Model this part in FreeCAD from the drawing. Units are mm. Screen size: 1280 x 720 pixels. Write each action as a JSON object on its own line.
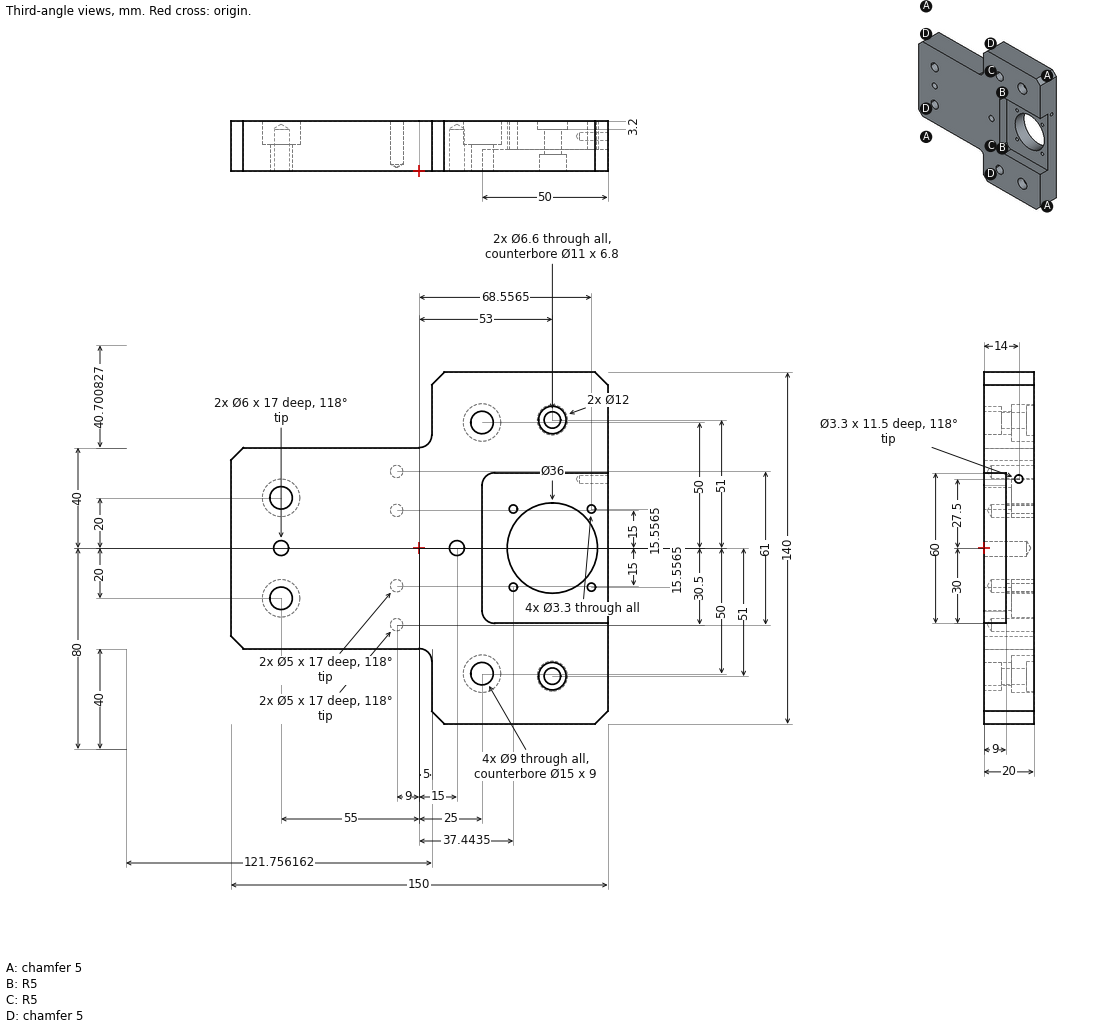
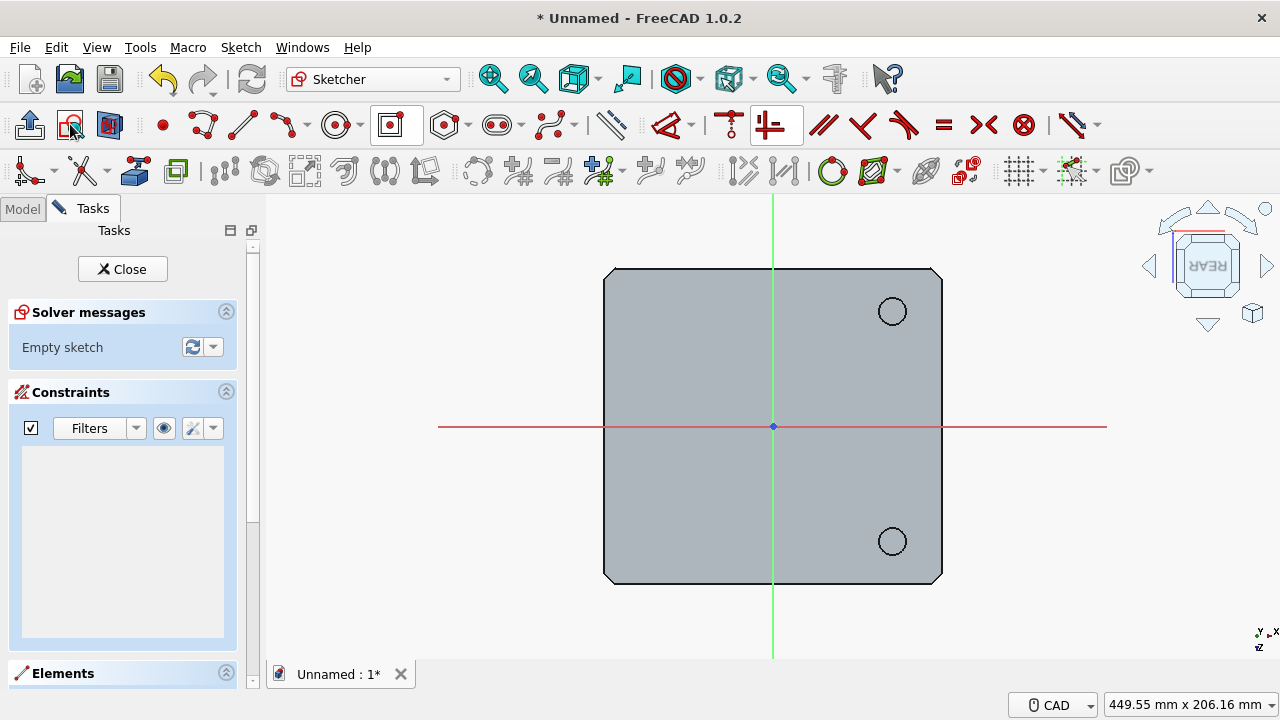
{"action": "scroll", "coordinate": [917, 426], "scroll_direction": "up", "scroll_amount": 6}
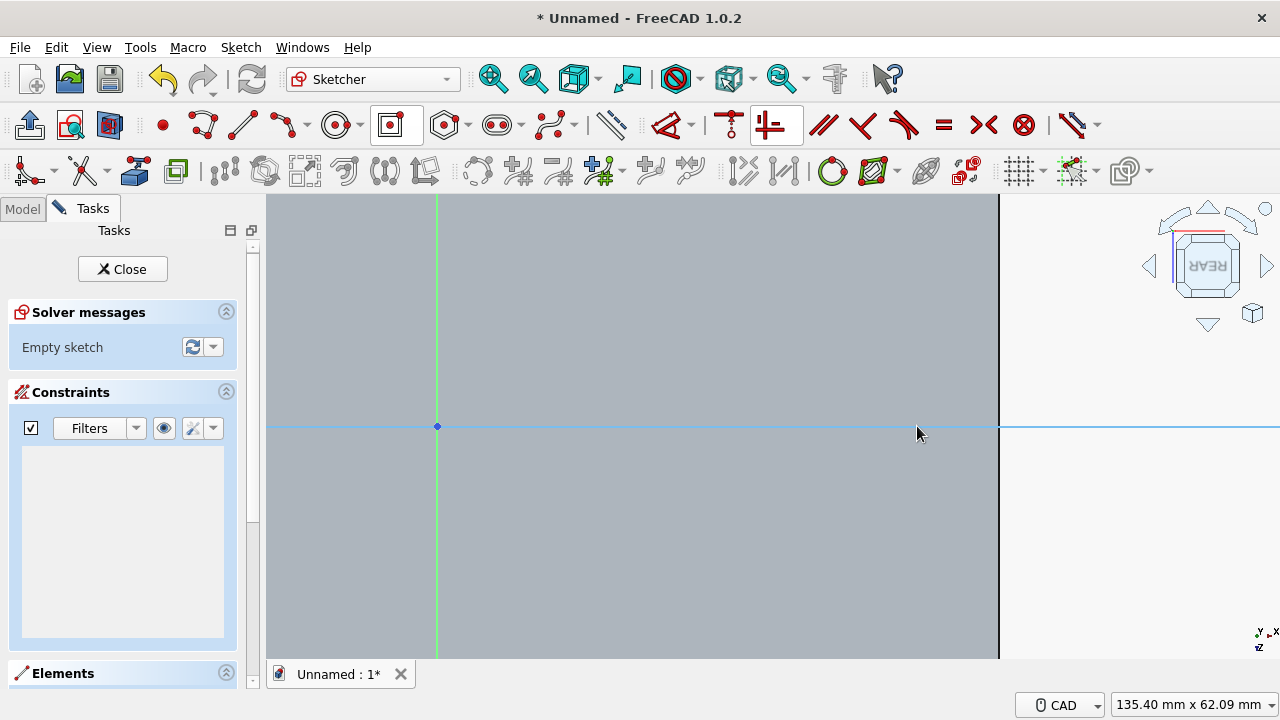
{"action": "left_click", "coordinate": [336, 126]}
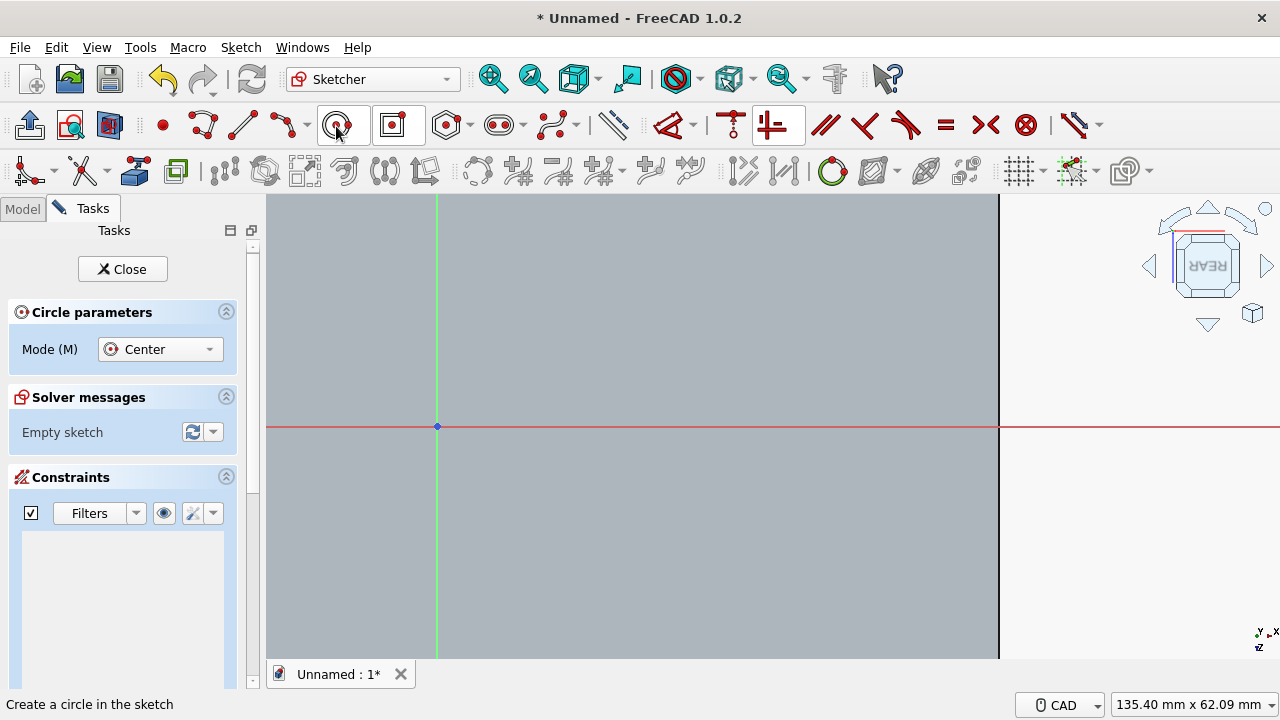
{"action": "left_click", "coordinate": [834, 426]}
{"action": "left_click", "coordinate": [930, 331]}
{"action": "key", "text": "Escape"}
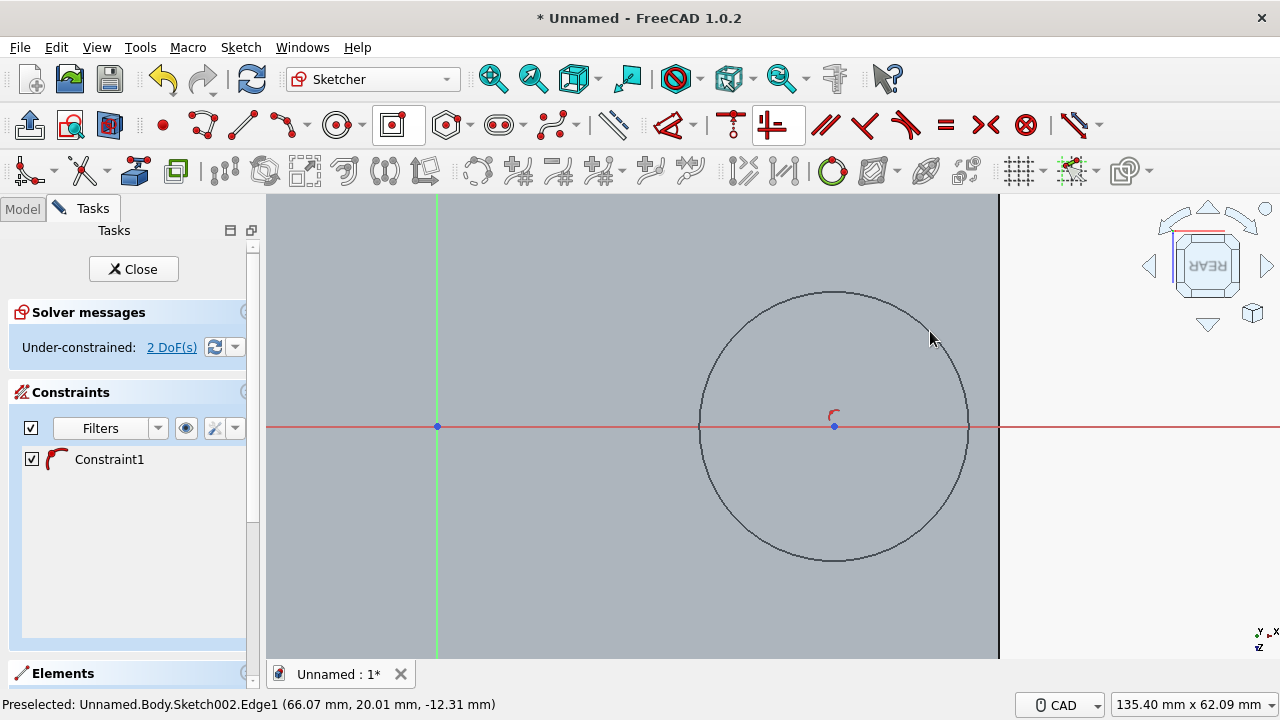
{"action": "left_click", "coordinate": [668, 126]}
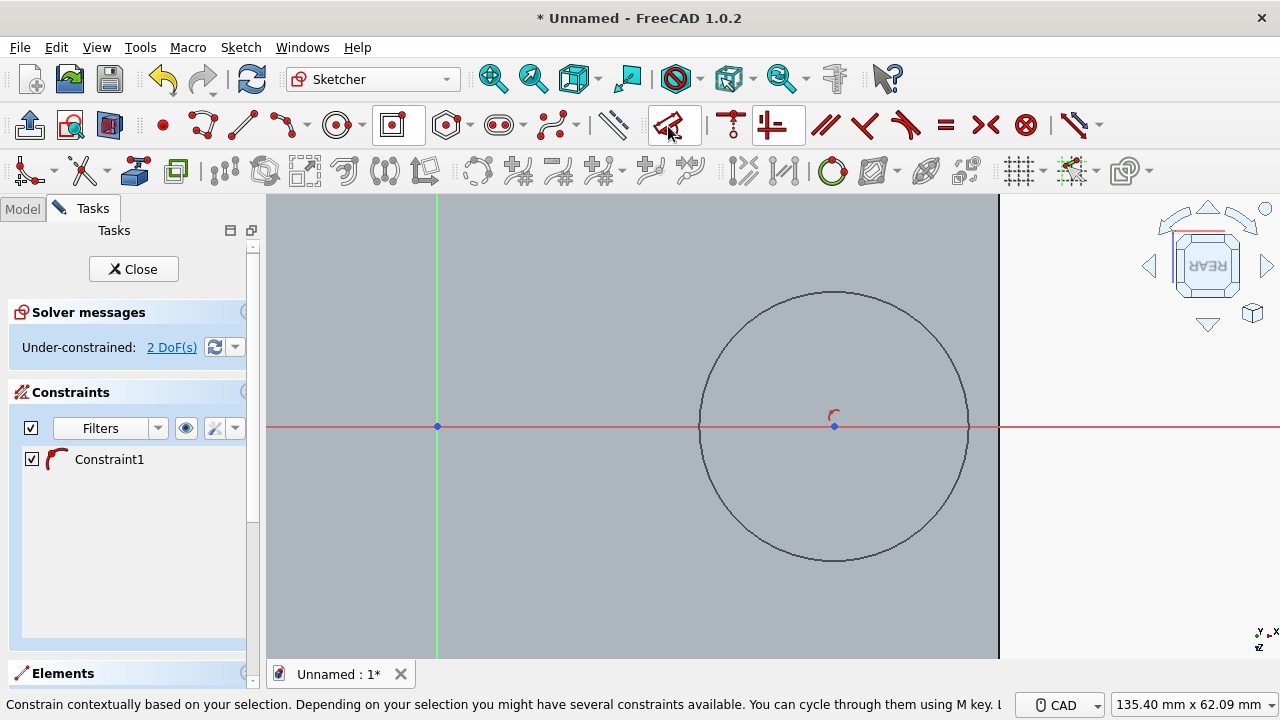
{"action": "left_click", "coordinate": [929, 331]}
{"action": "left_click", "coordinate": [952, 308]}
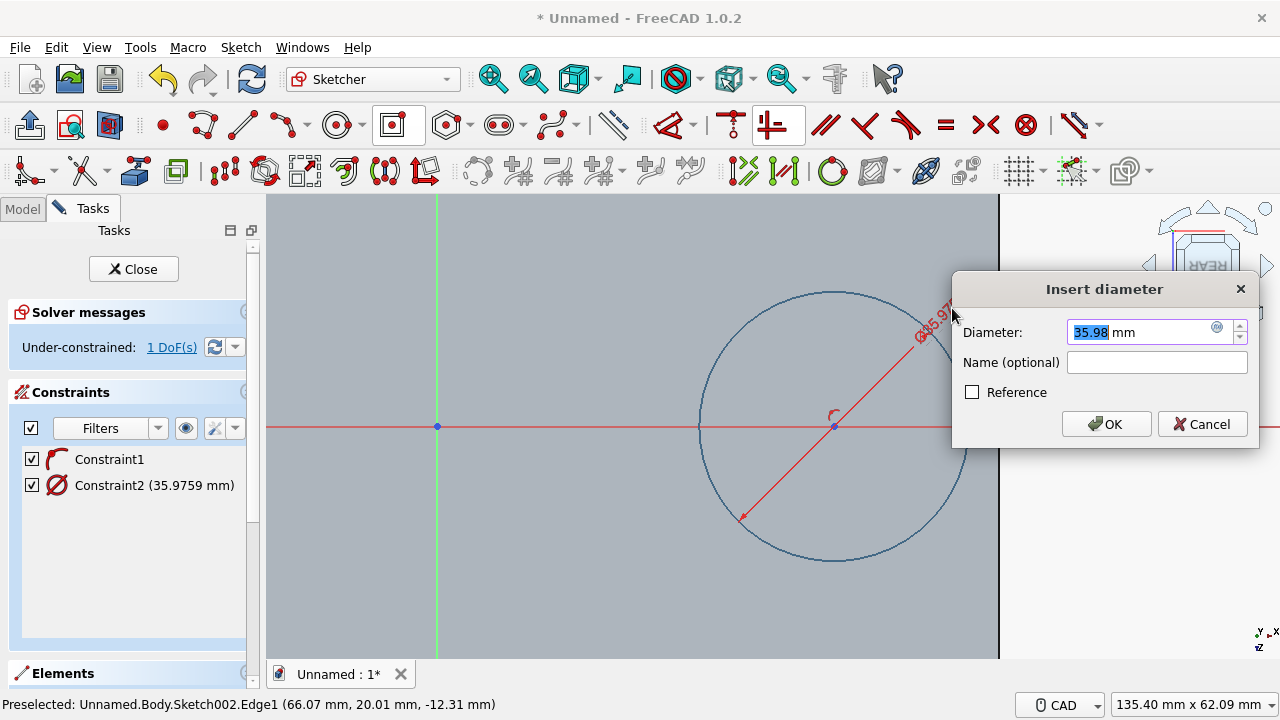
{"action": "type", "text": "36"}
{"action": "key", "text": "Return"}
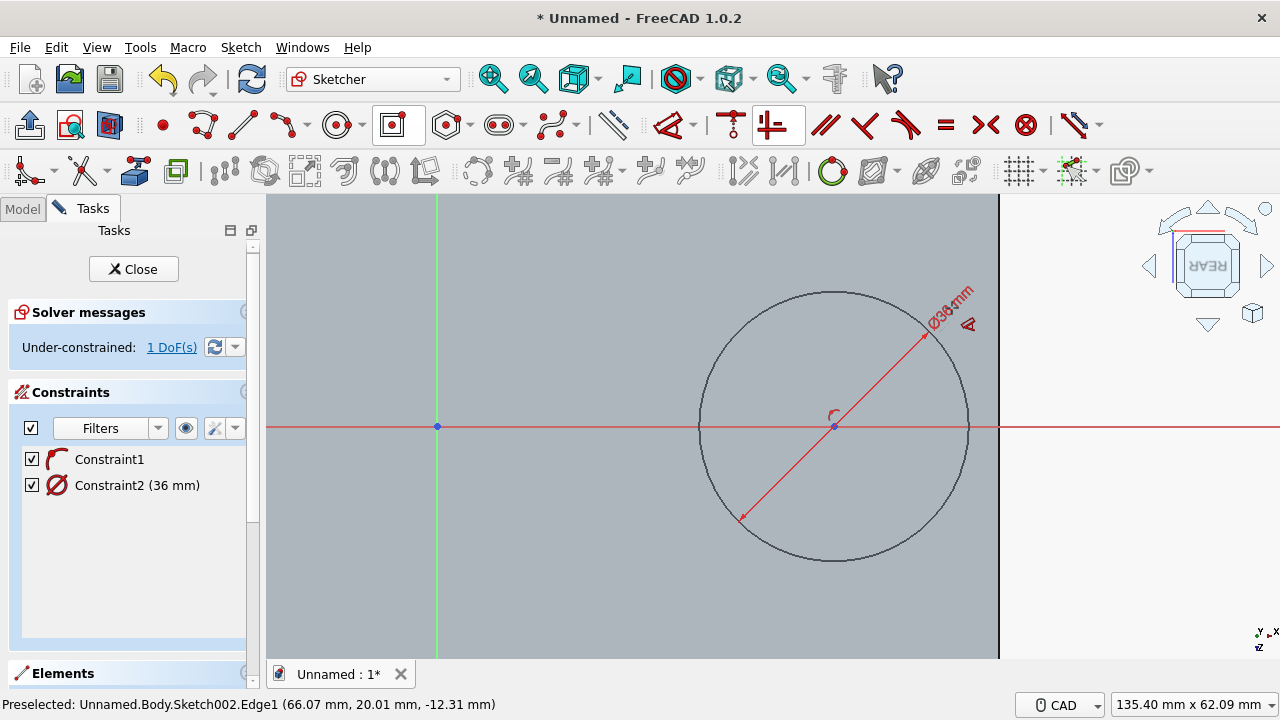
{"action": "left_click", "coordinate": [834, 426]}
{"action": "left_click", "coordinate": [636, 460]}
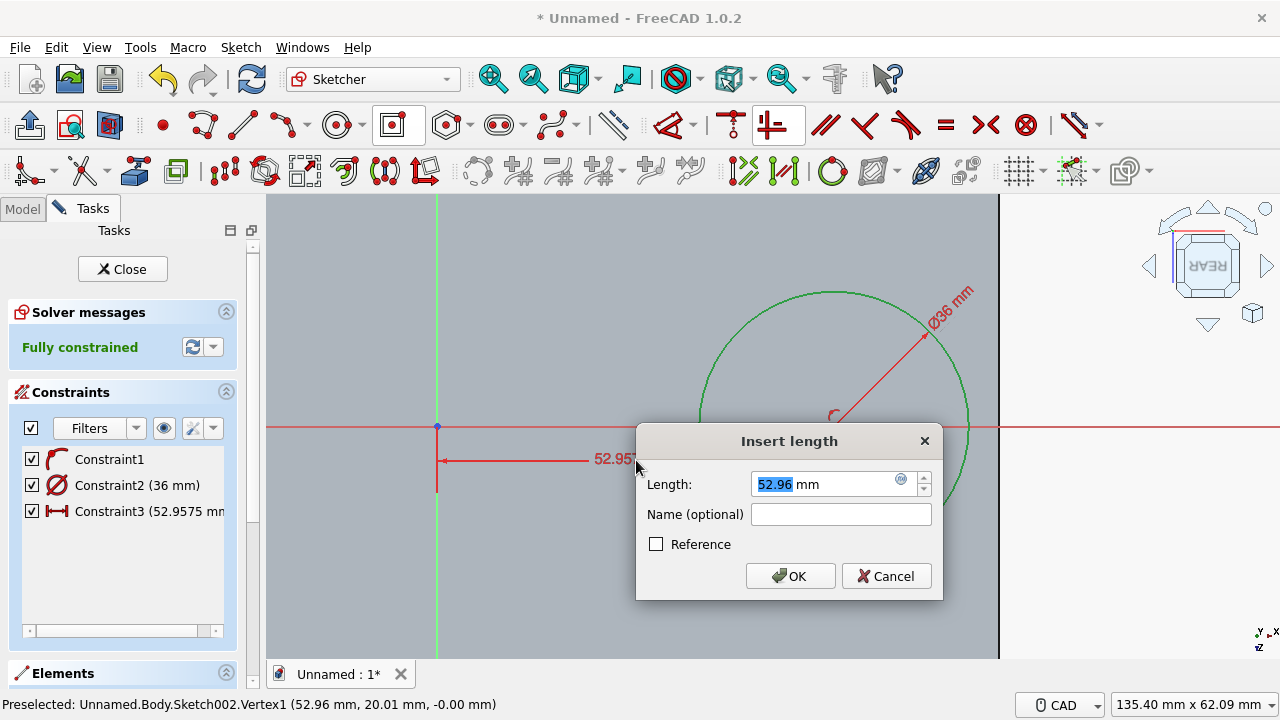
{"action": "type", "text": "53"}
{"action": "key", "text": "Return"}
{"action": "key", "text": "Escape"}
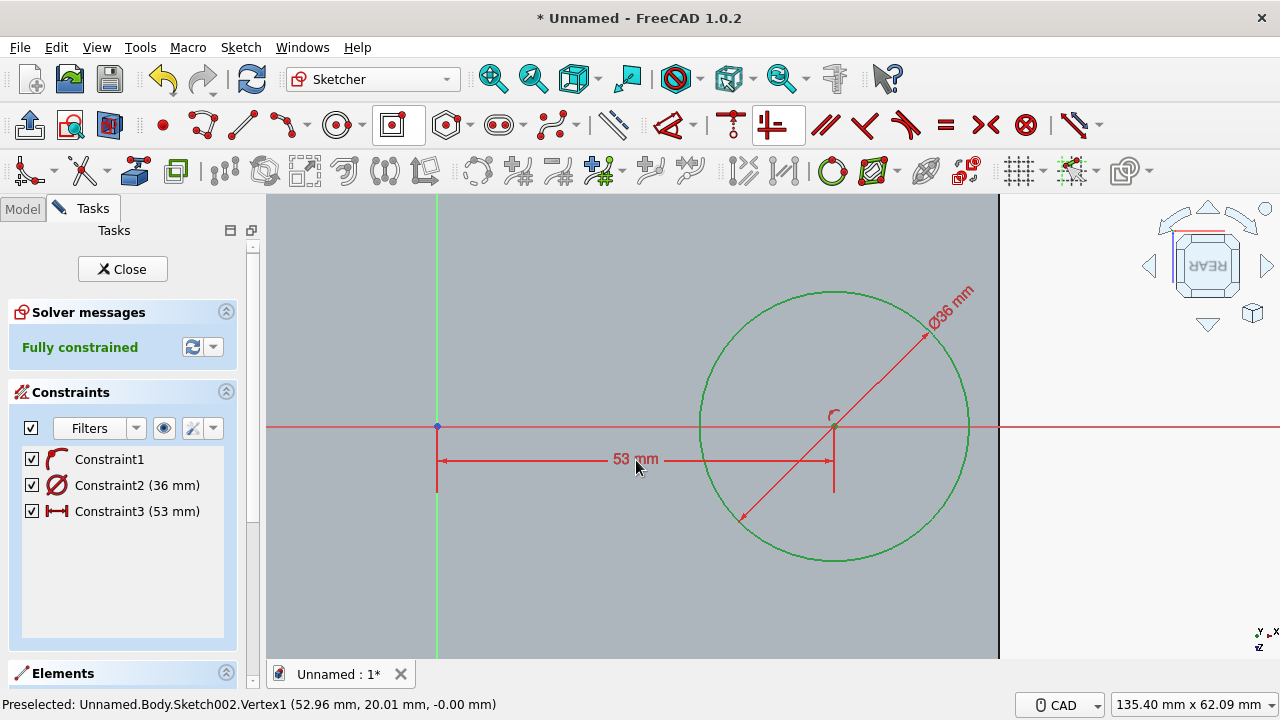
{"action": "left_click", "coordinate": [123, 269]}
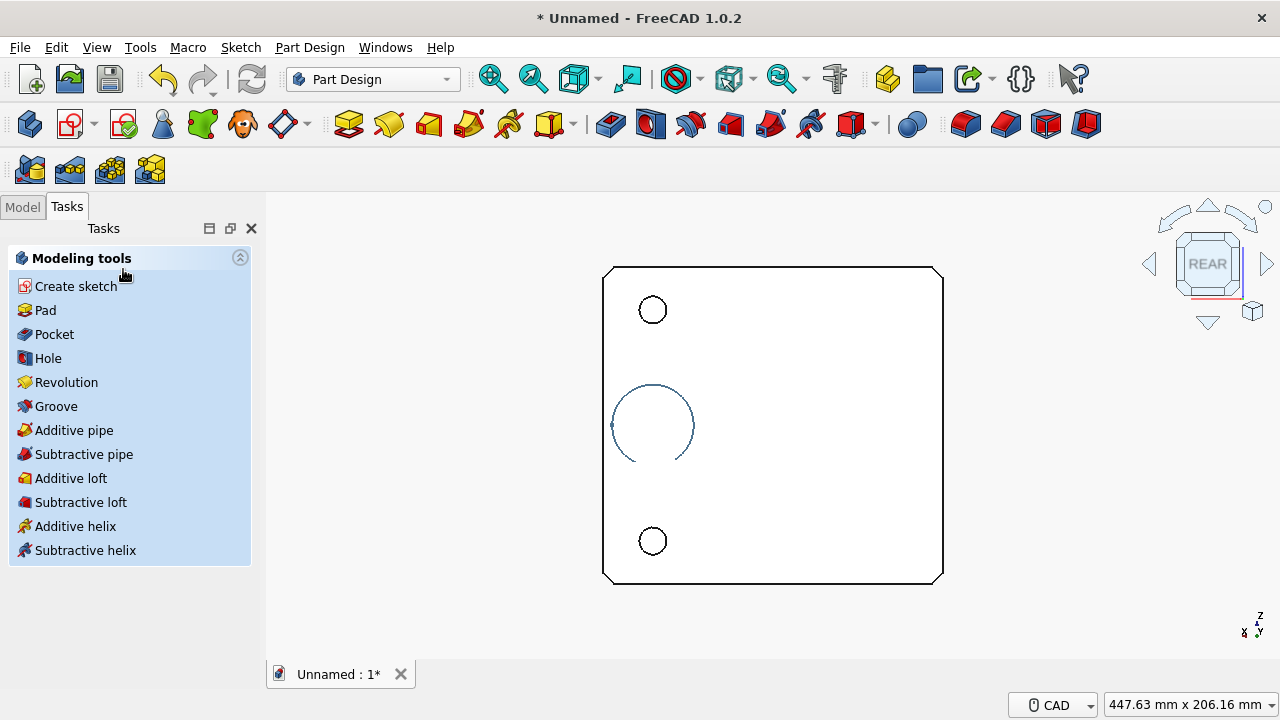
{"action": "left_click", "coordinate": [612, 124]}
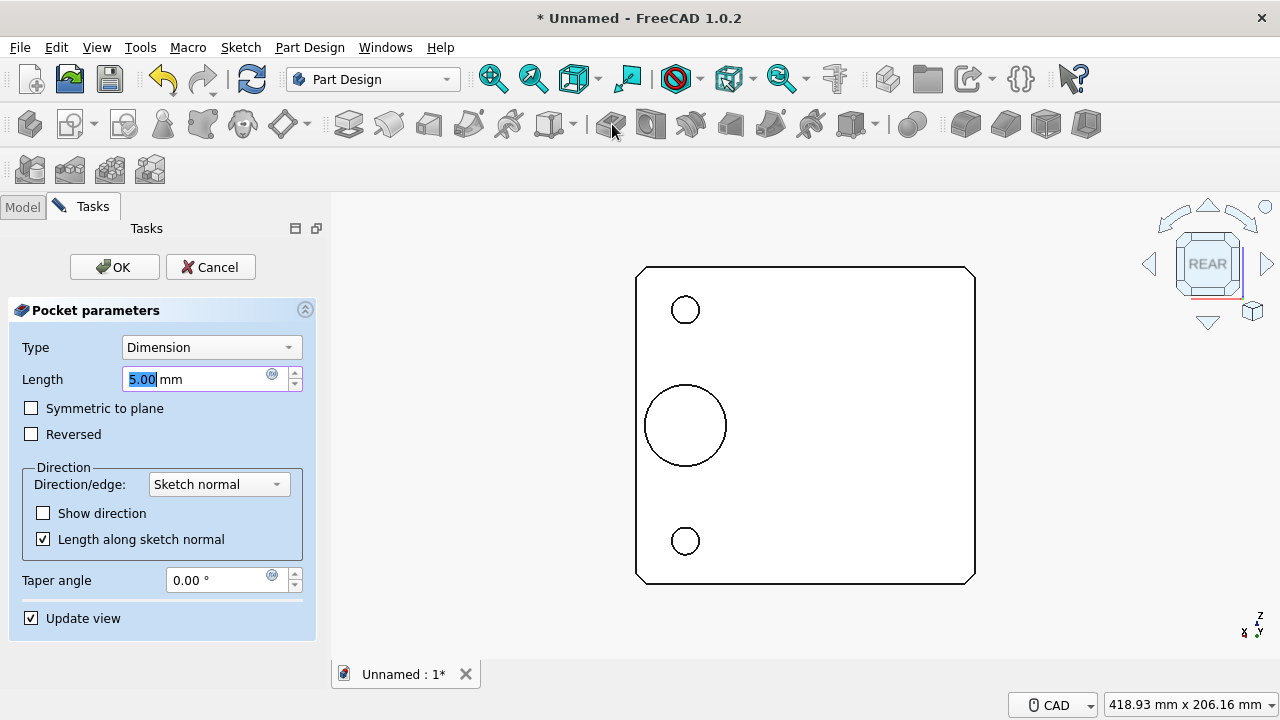
{"action": "left_click", "coordinate": [212, 348]}